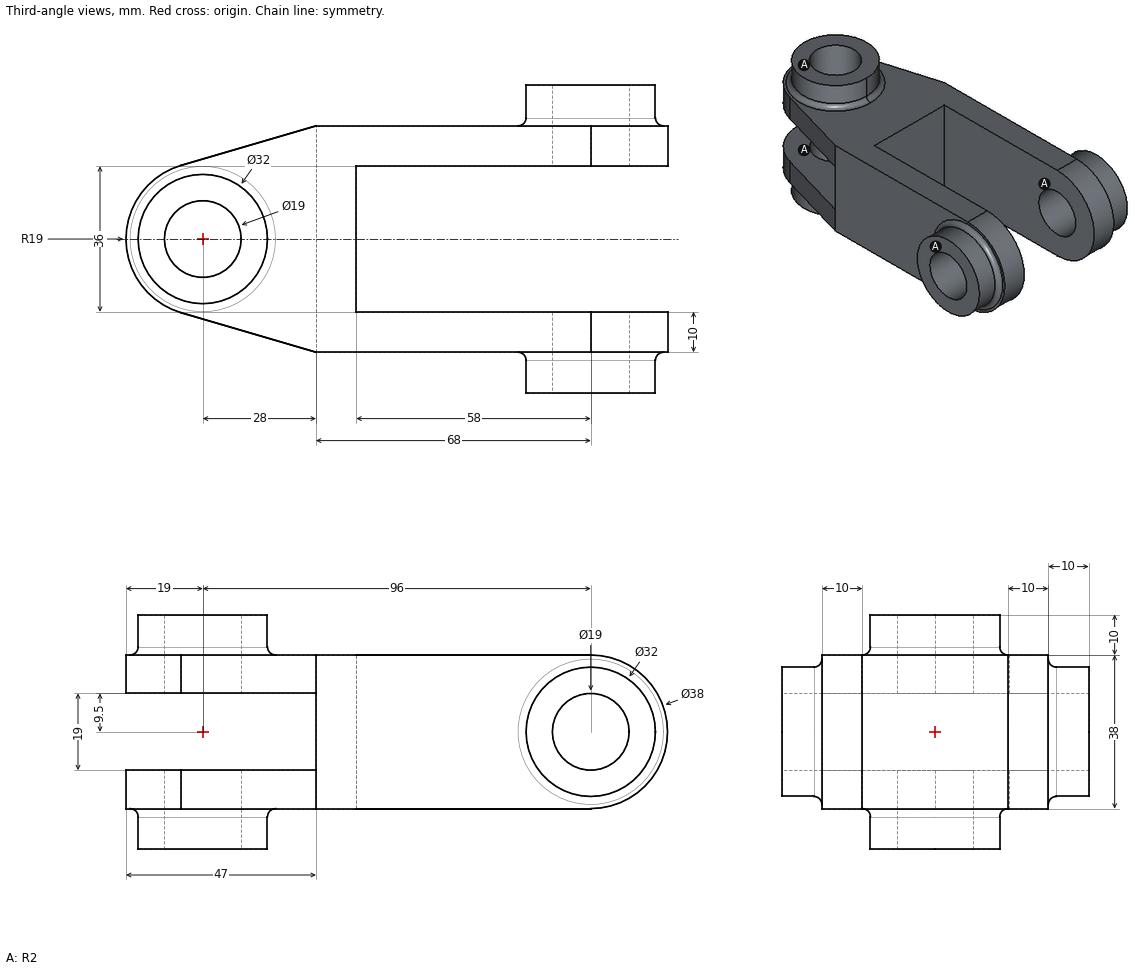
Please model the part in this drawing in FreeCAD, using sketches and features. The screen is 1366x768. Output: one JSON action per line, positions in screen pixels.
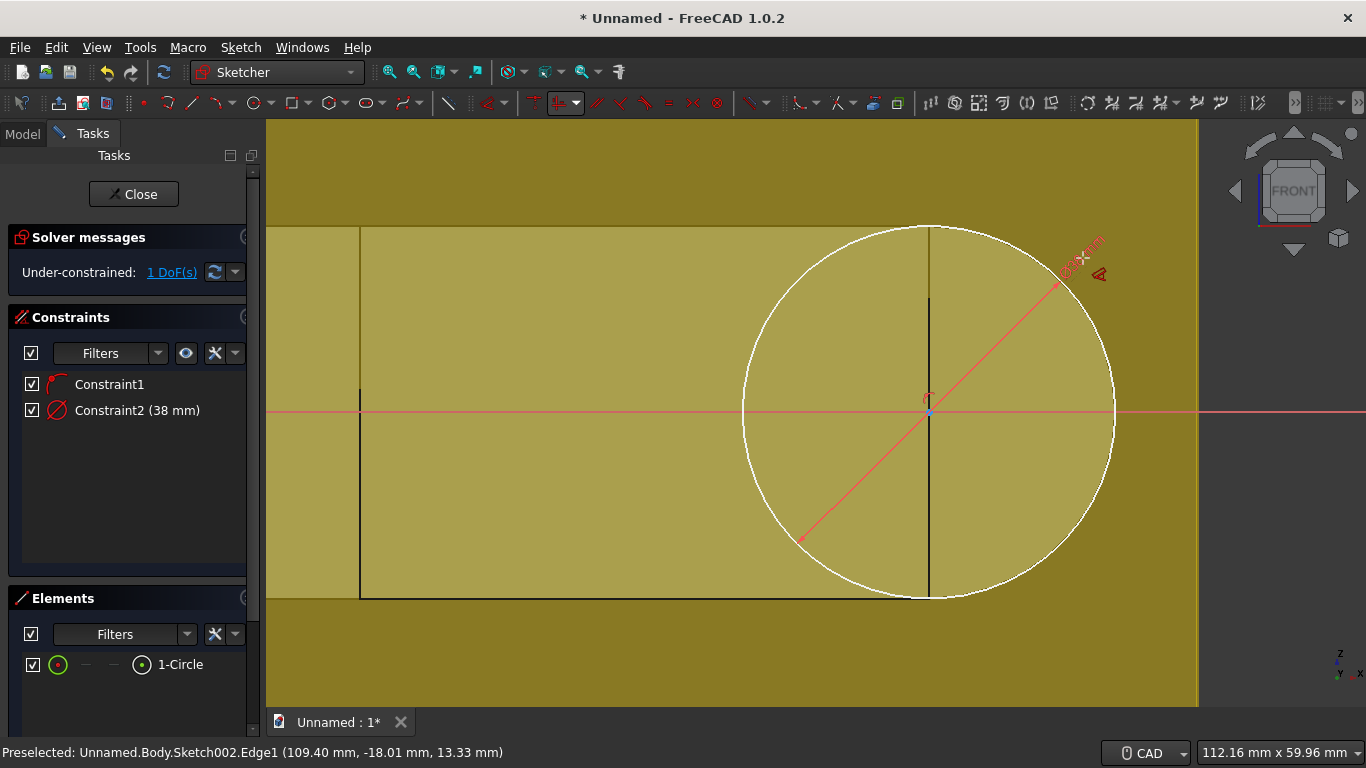
{"action": "left_click", "coordinate": [929, 412]}
{"action": "left_click", "coordinate": [612, 446]}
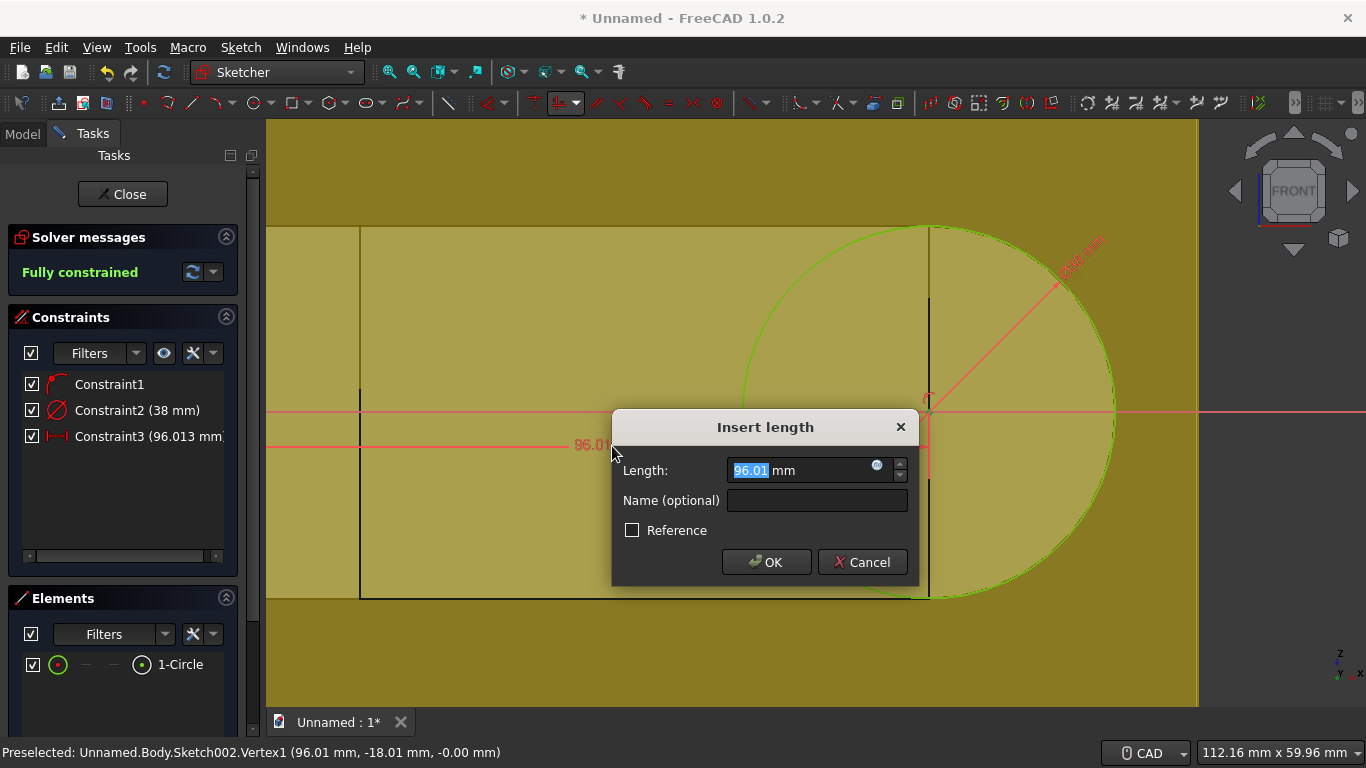
{"action": "type", "text": "96"}
{"action": "key", "text": "Return"}
{"action": "key", "text": "Escape"}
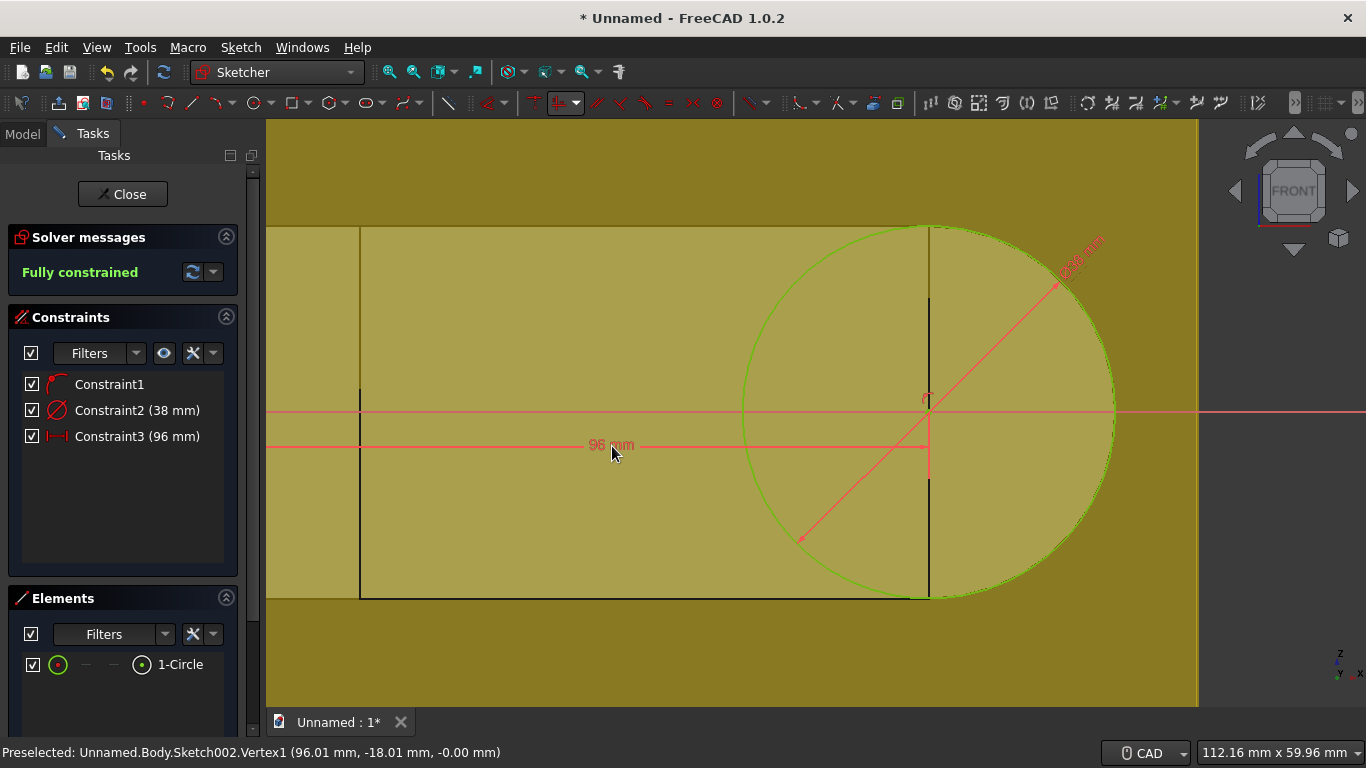
{"action": "left_click", "coordinate": [123, 194]}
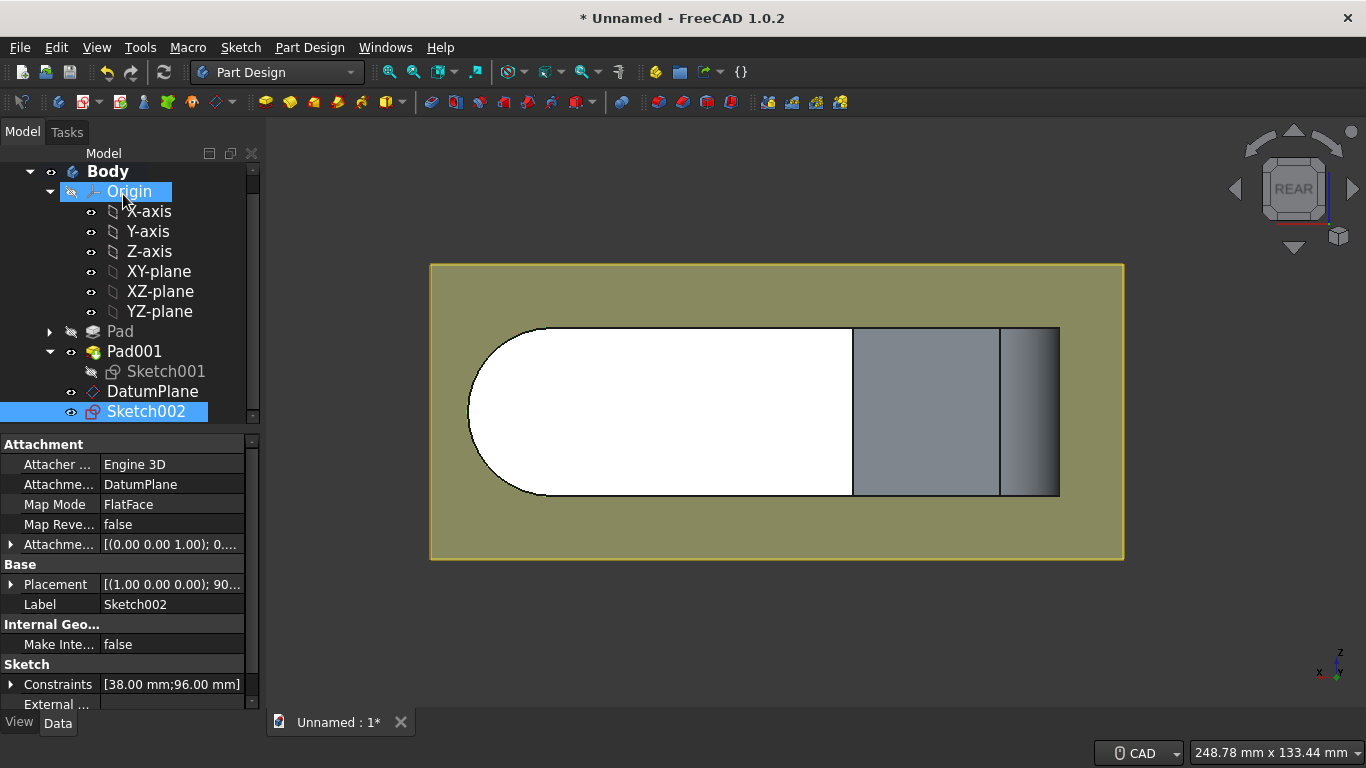
{"action": "left_click", "coordinate": [266, 102]}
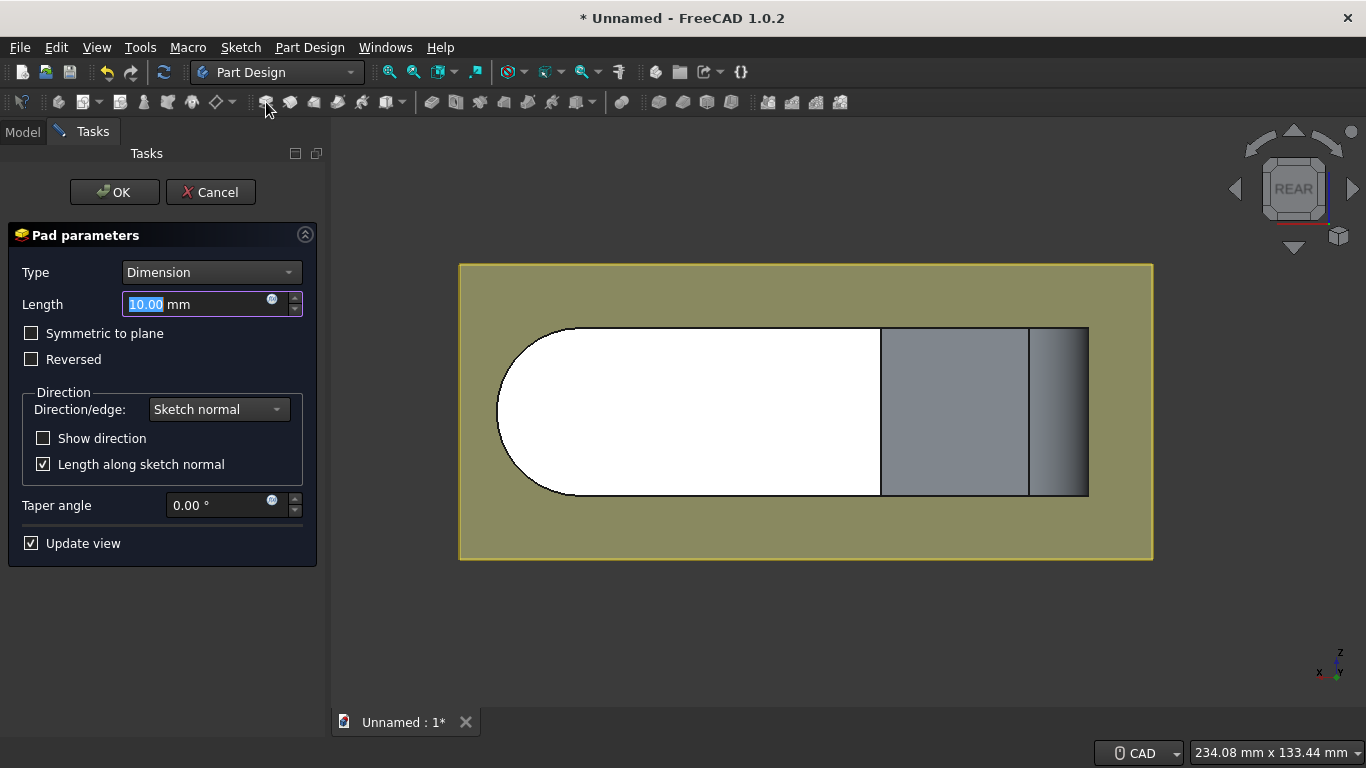
{"action": "type", "text": "10"}
{"action": "key", "text": "Tab"}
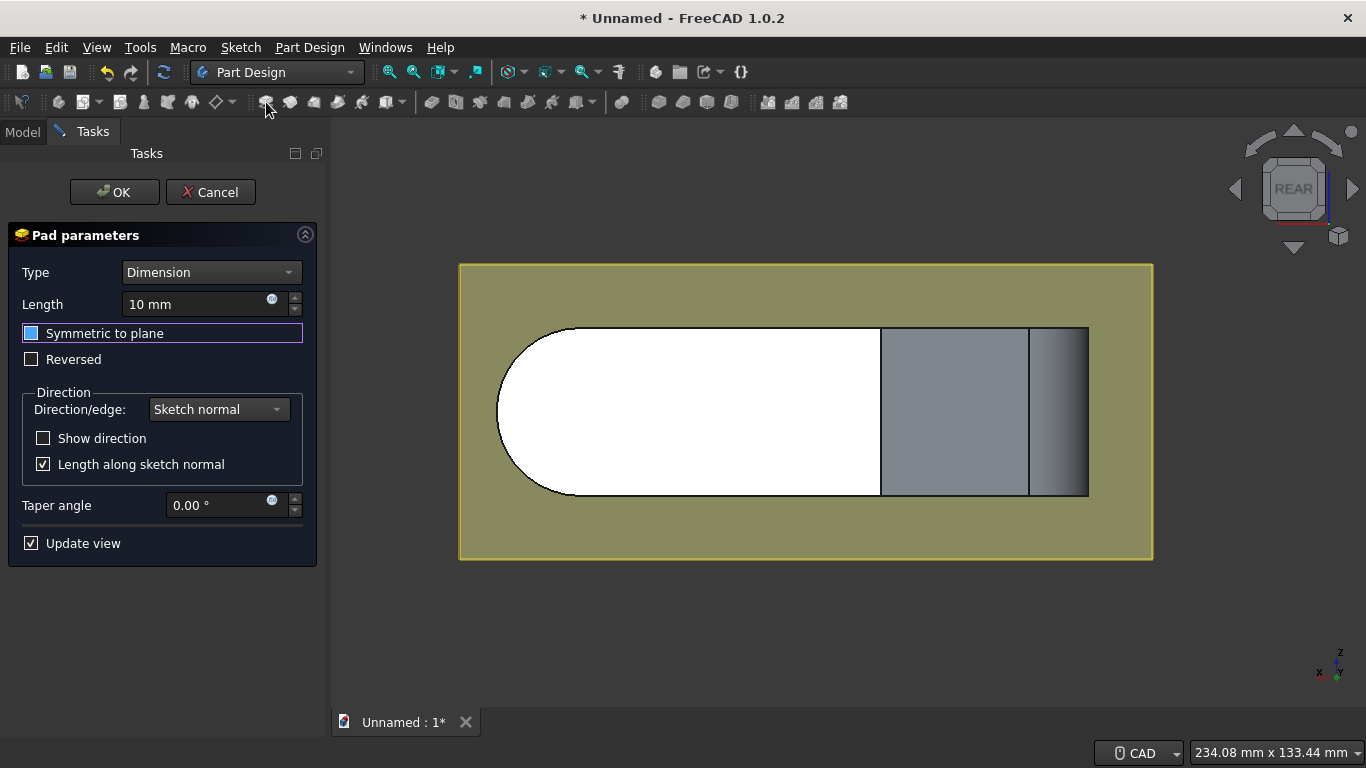
{"action": "left_click", "coordinate": [115, 192]}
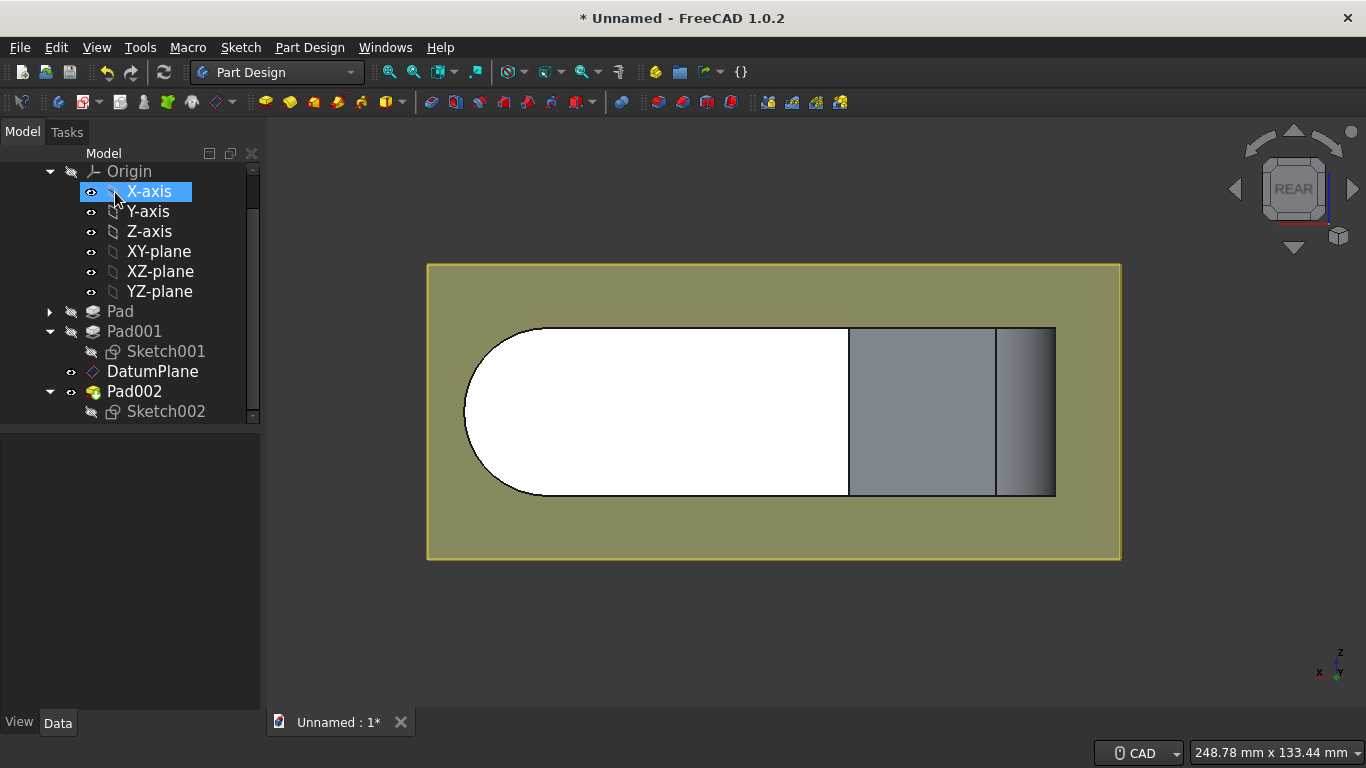
{"action": "left_click", "coordinate": [116, 372]}
{"action": "key", "text": "space"}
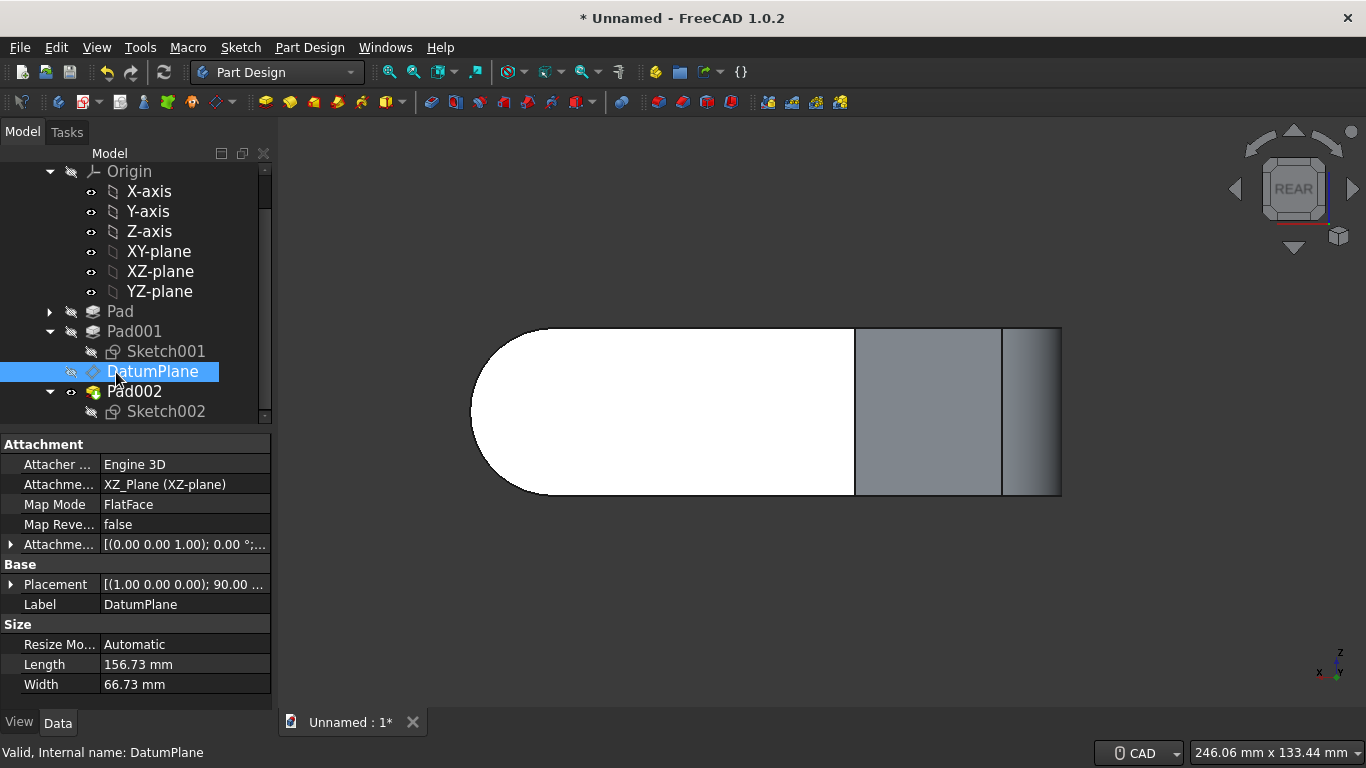
{"action": "key", "text": "0"}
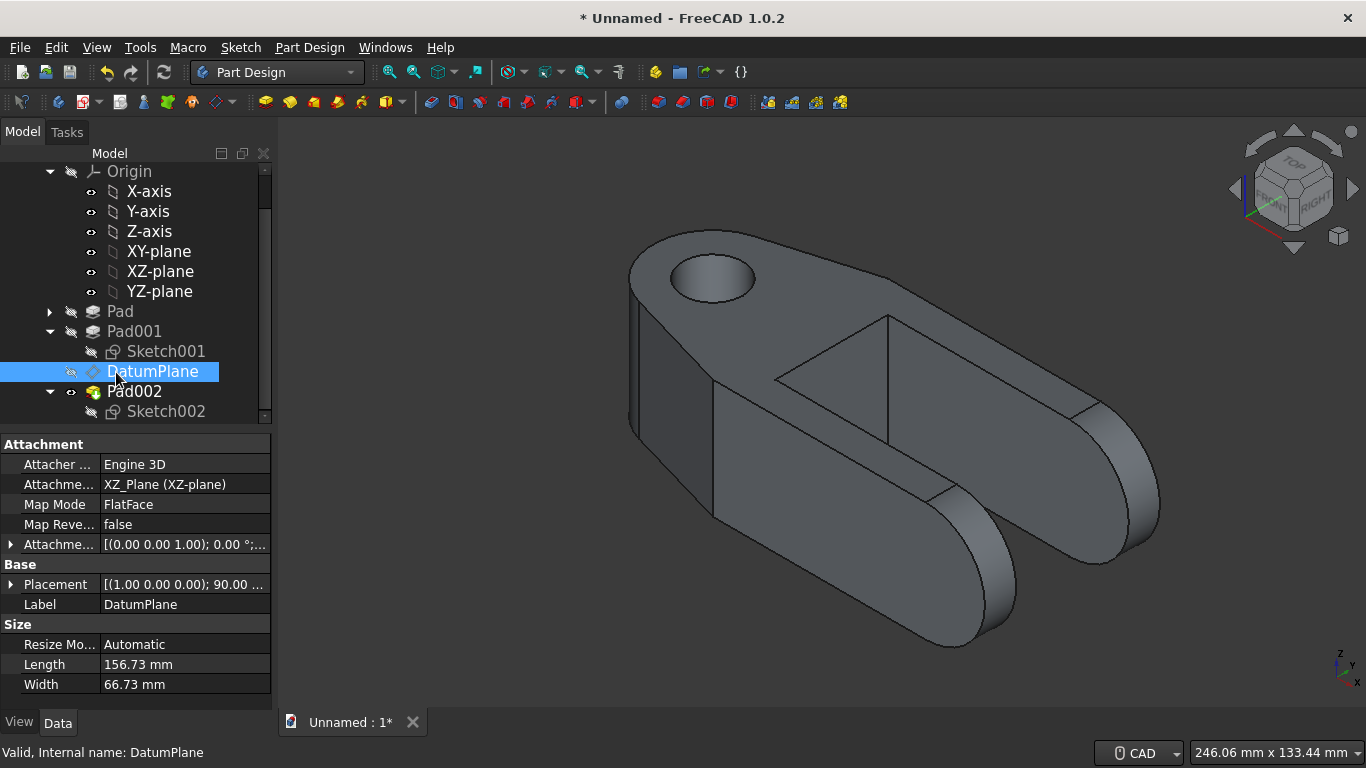
{"action": "left_click", "coordinate": [888, 548]}